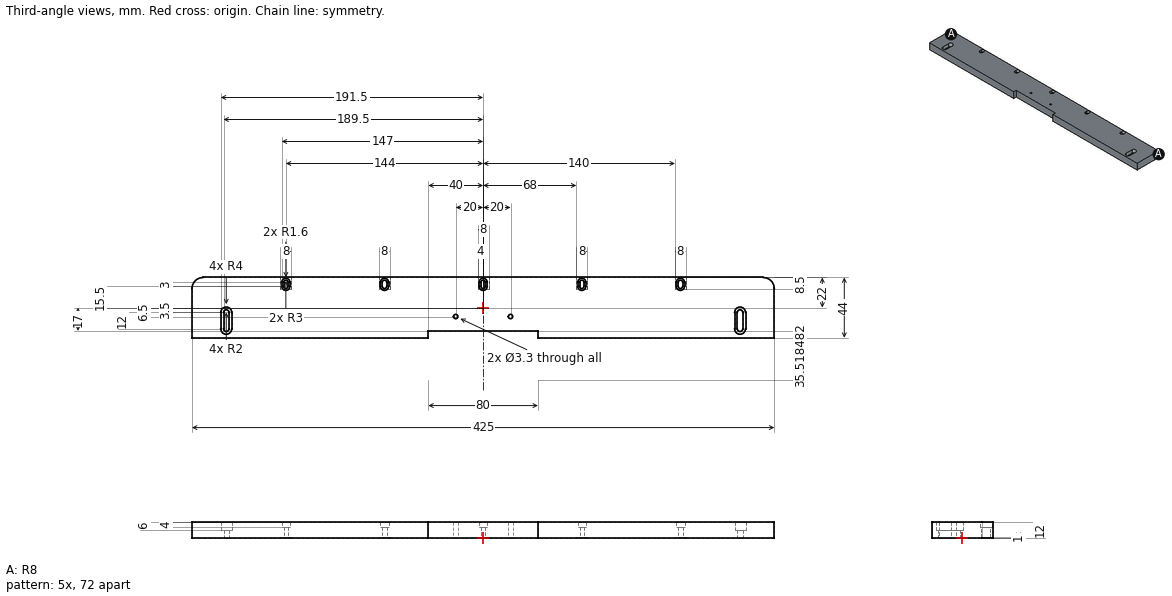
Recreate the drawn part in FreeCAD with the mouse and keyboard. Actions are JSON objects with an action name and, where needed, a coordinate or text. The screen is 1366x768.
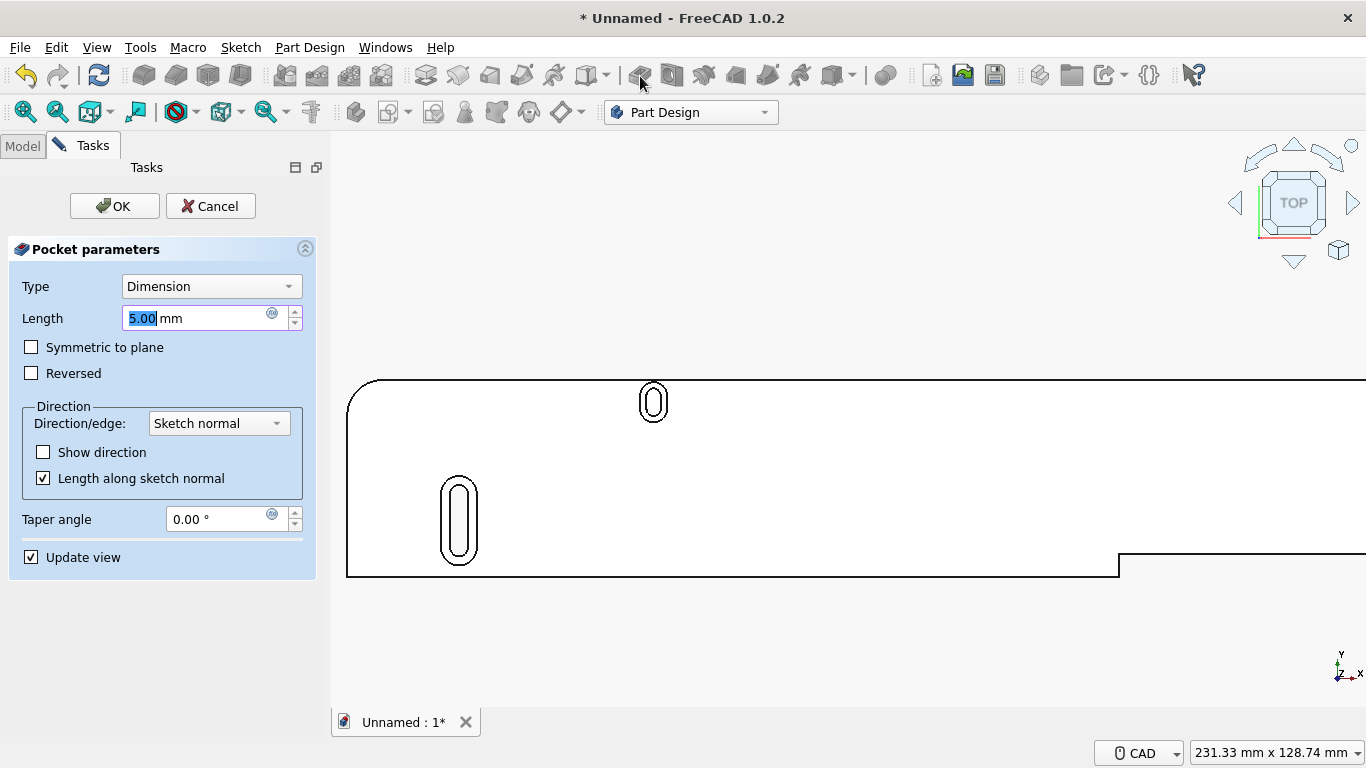
{"action": "left_click", "coordinate": [212, 286]}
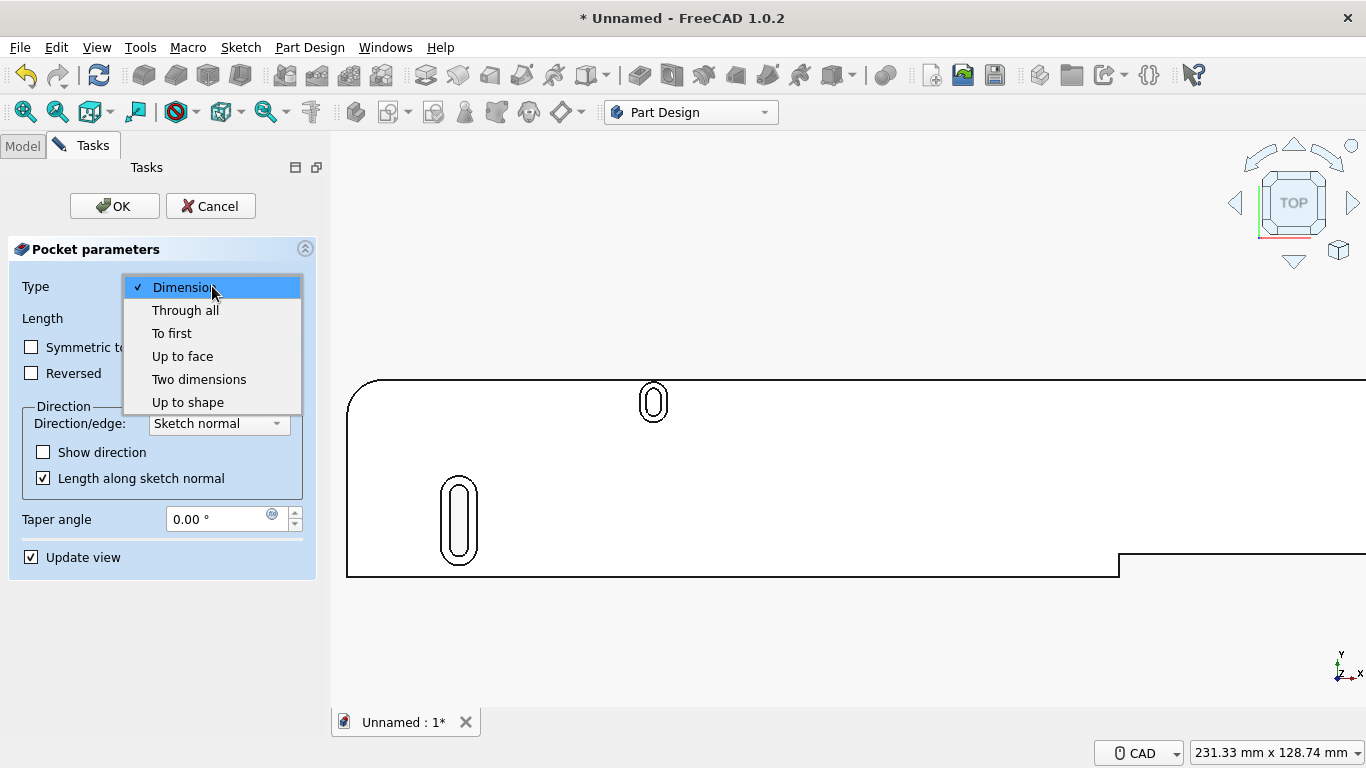
{"action": "left_click", "coordinate": [212, 310]}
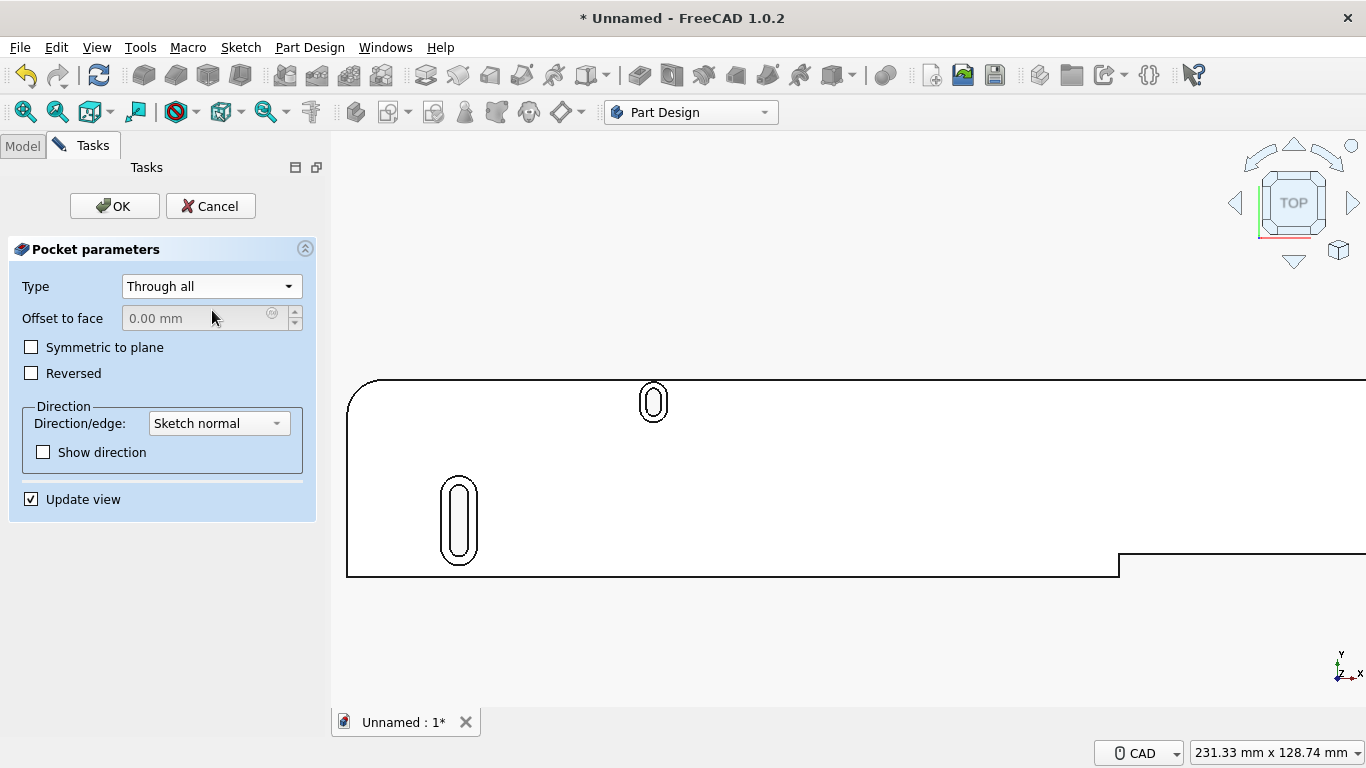
{"action": "left_click", "coordinate": [115, 206]}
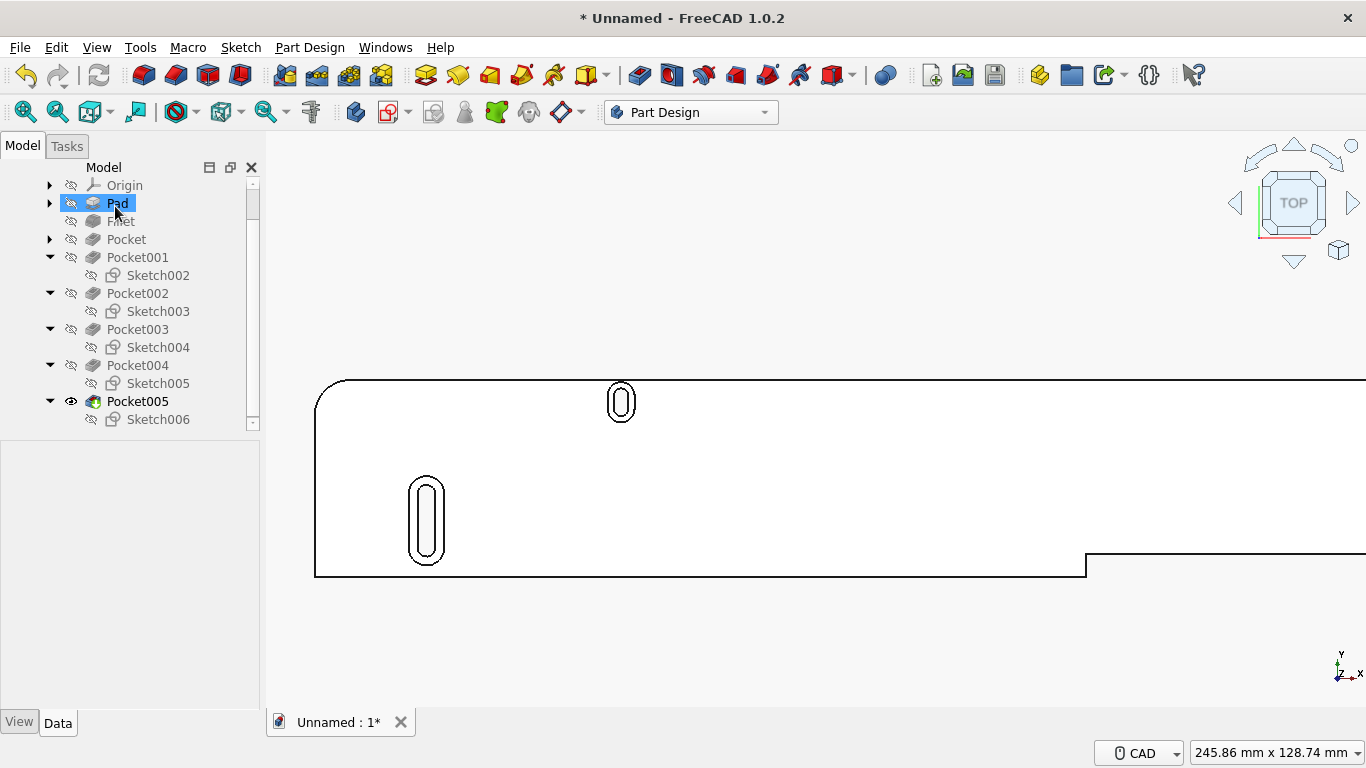
{"action": "left_click", "coordinate": [26, 112]}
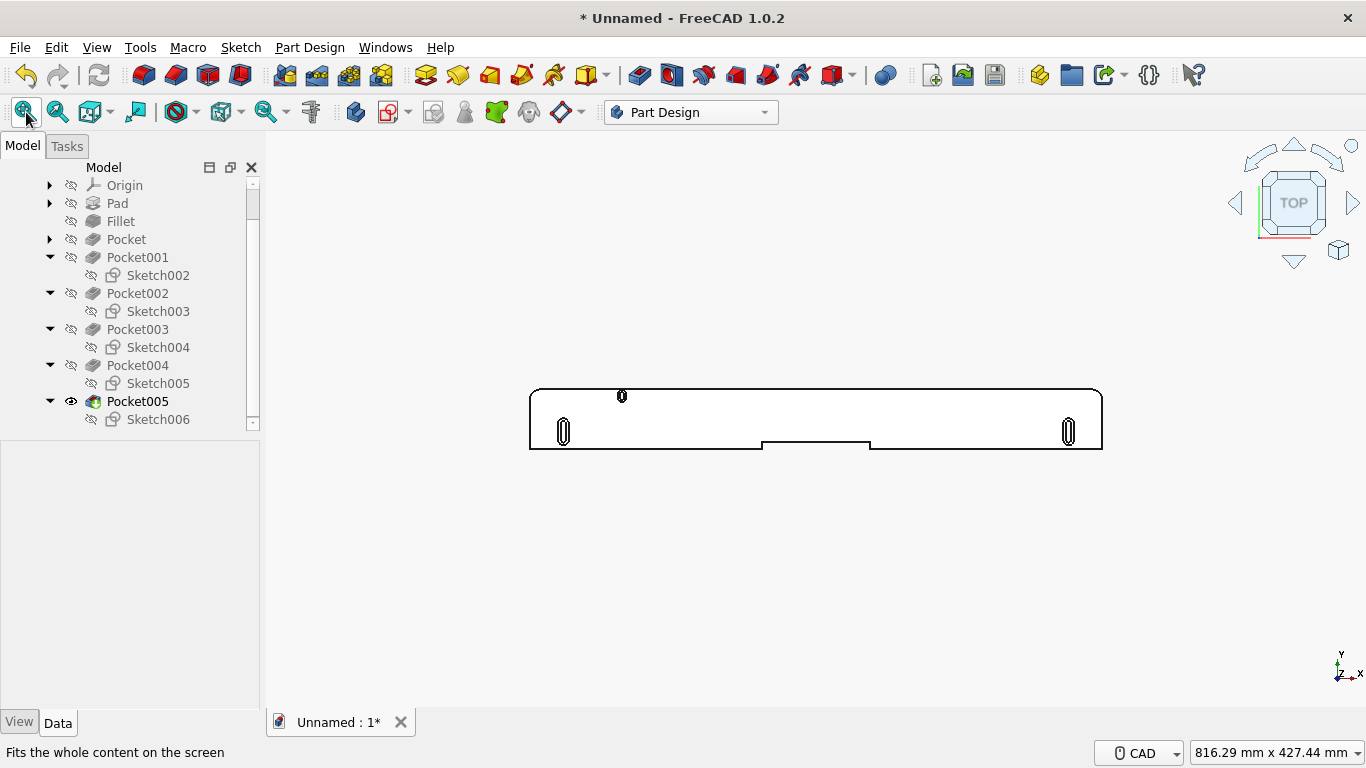
{"action": "left_click", "coordinate": [116, 365]}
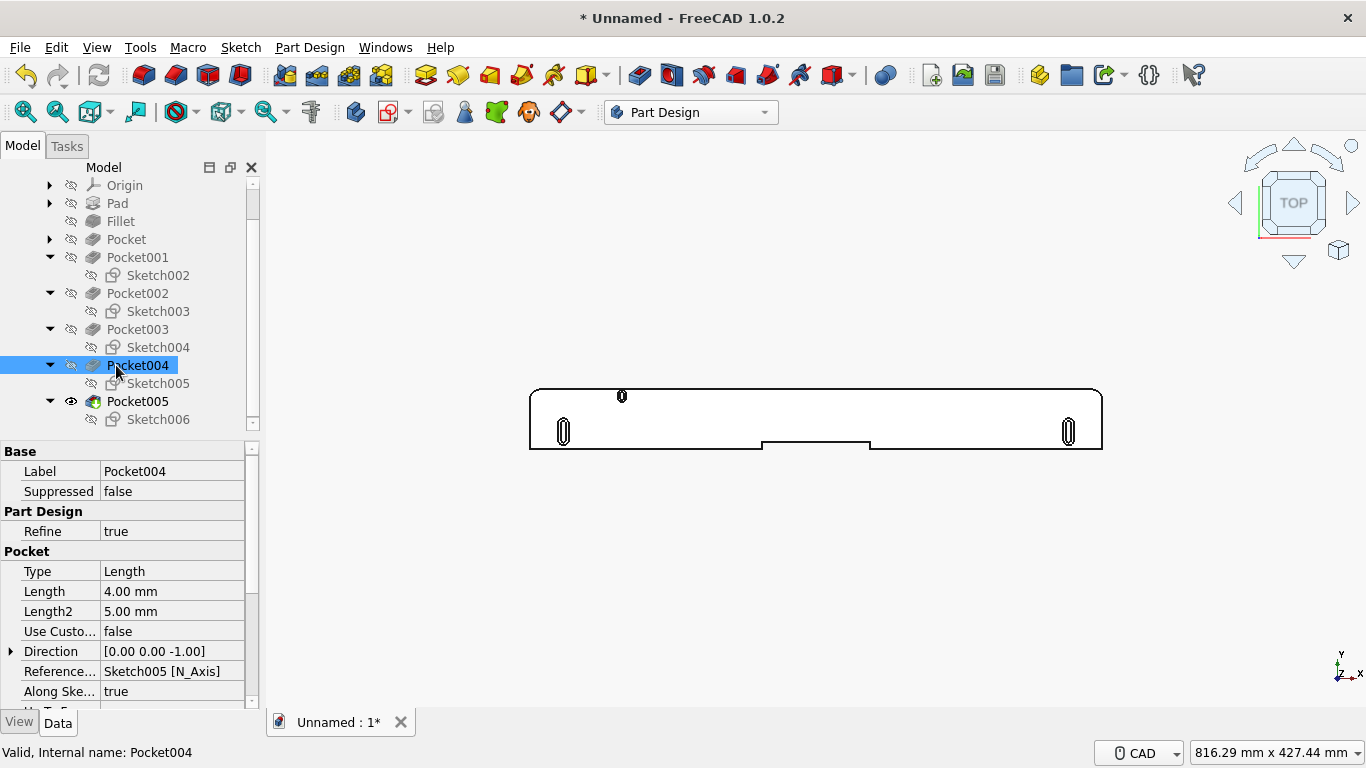
{"action": "left_click", "coordinate": [116, 401], "text": "ctrl"}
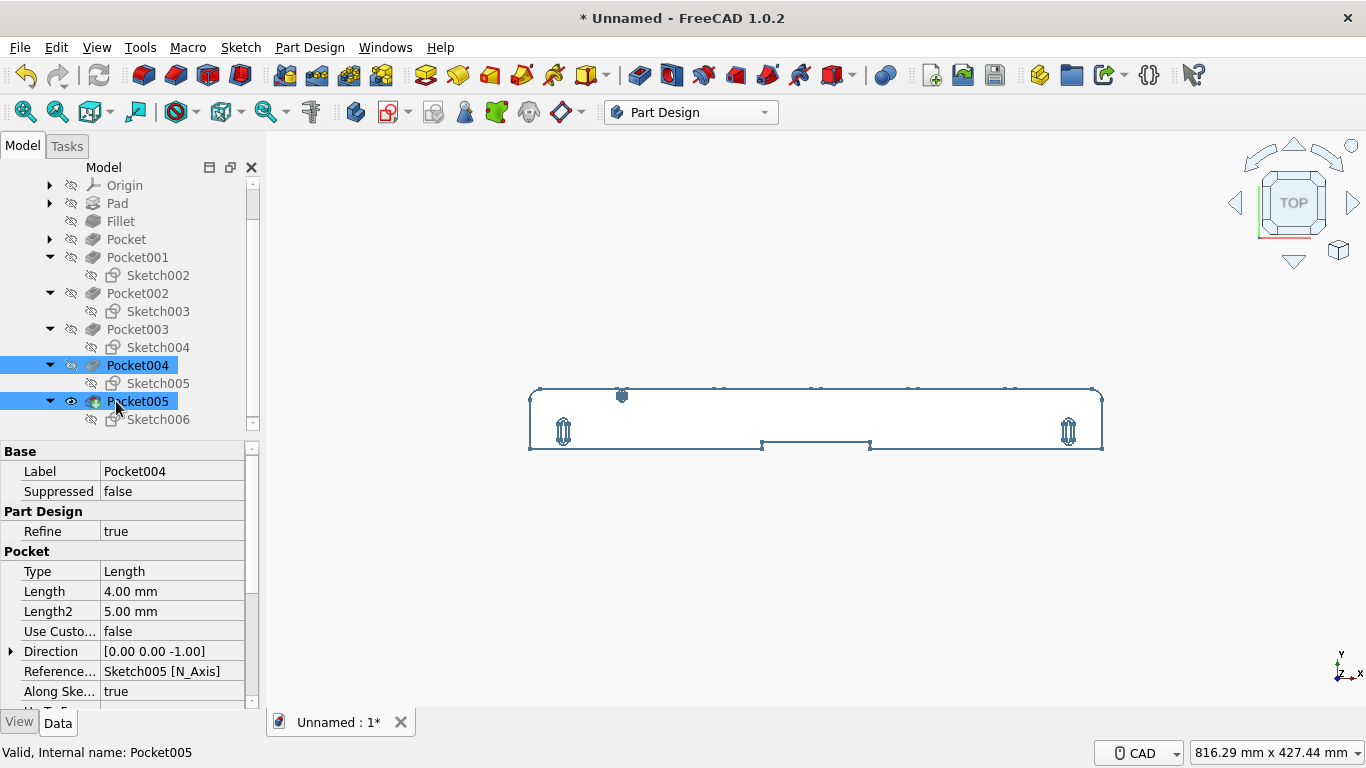
{"action": "left_click", "coordinate": [318, 76]}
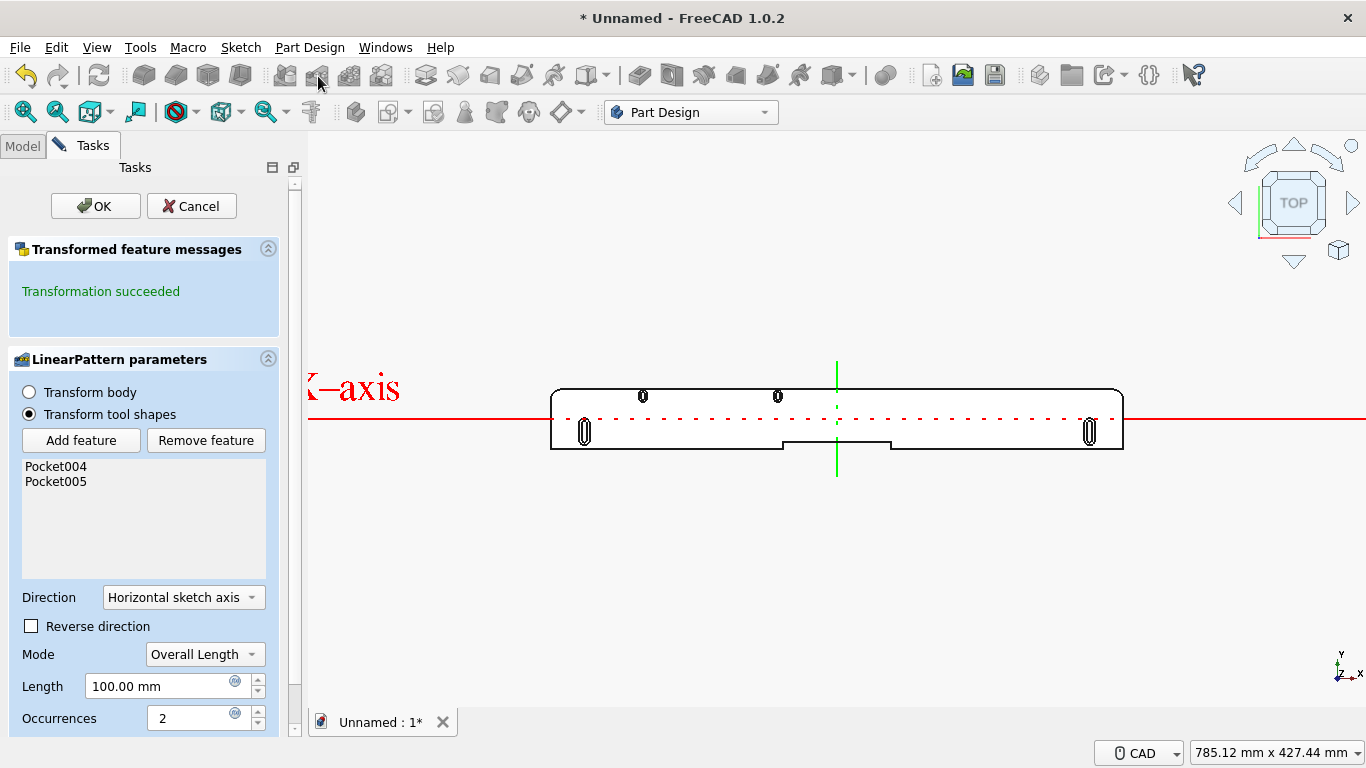
{"action": "left_click", "coordinate": [184, 598]}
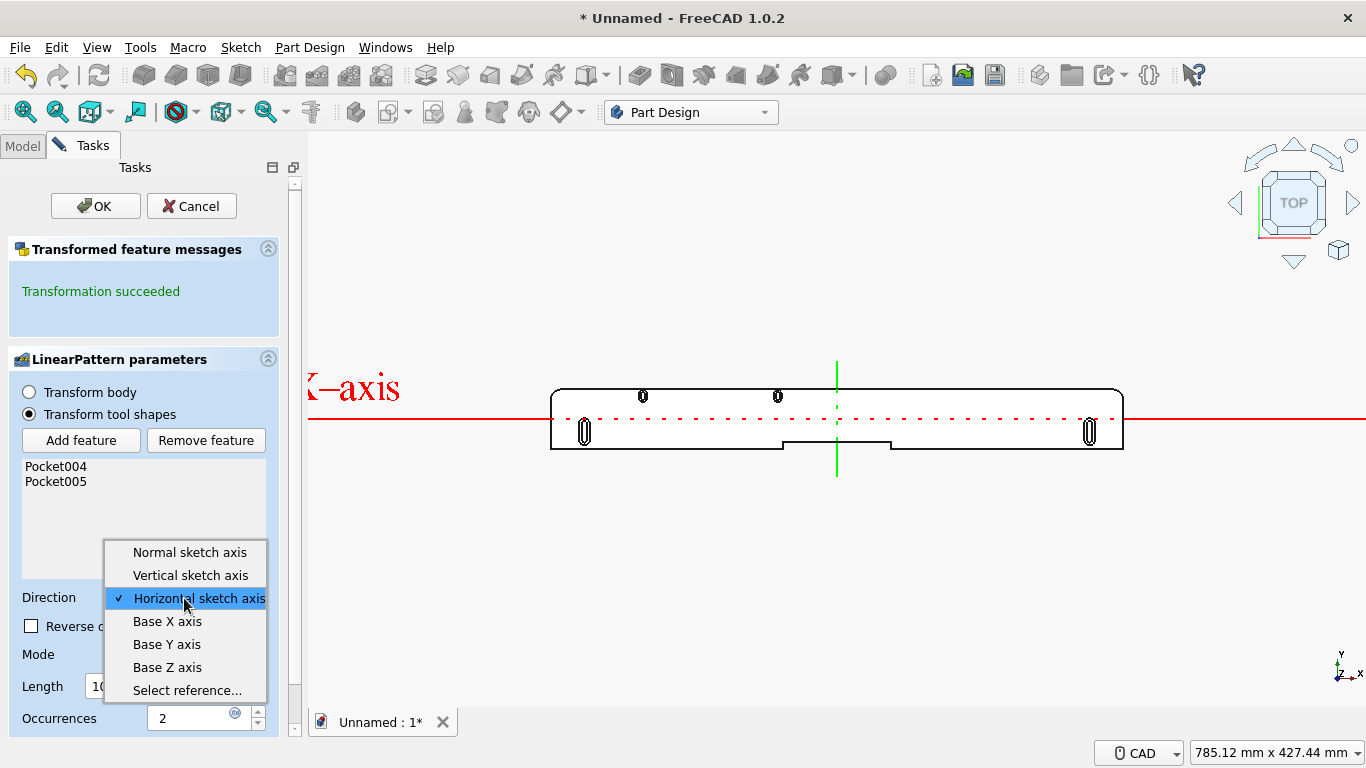
{"action": "left_click", "coordinate": [184, 622]}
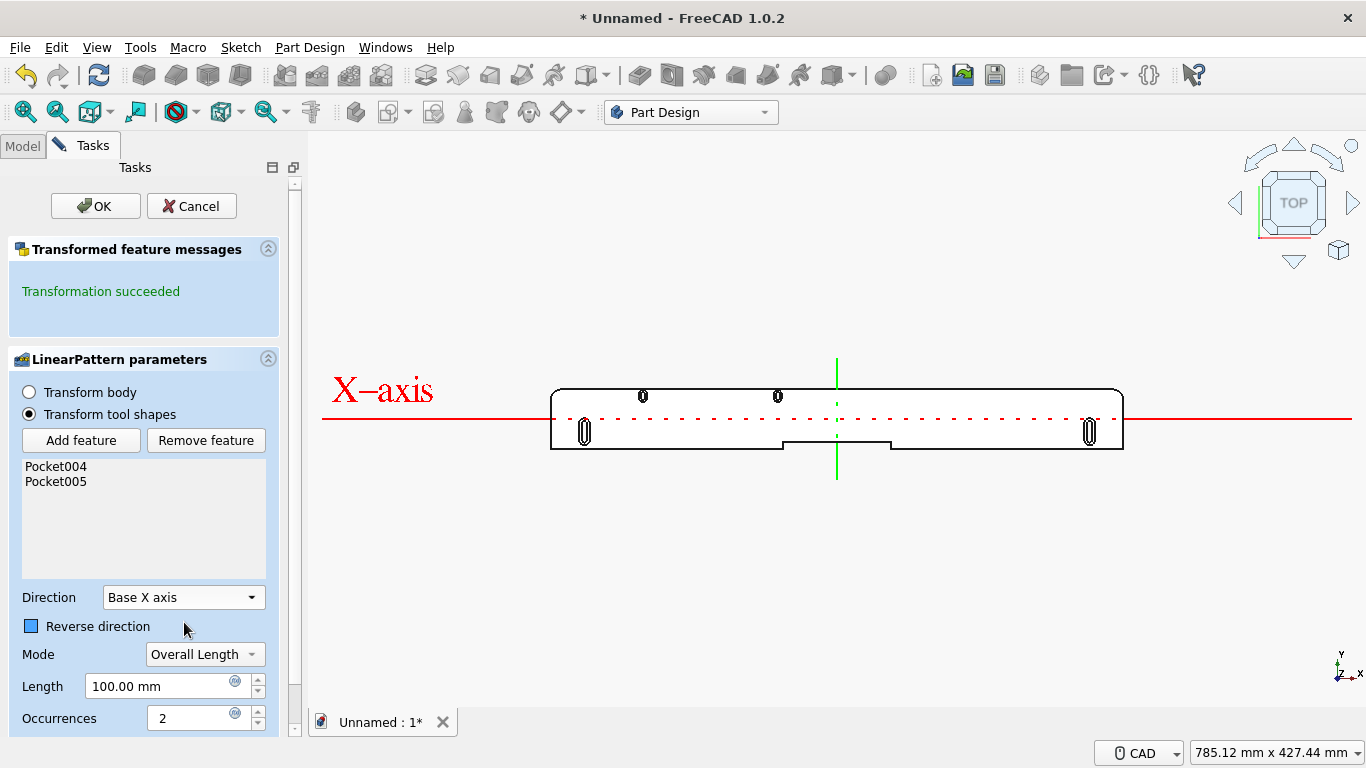
{"action": "left_click", "coordinate": [206, 654]}